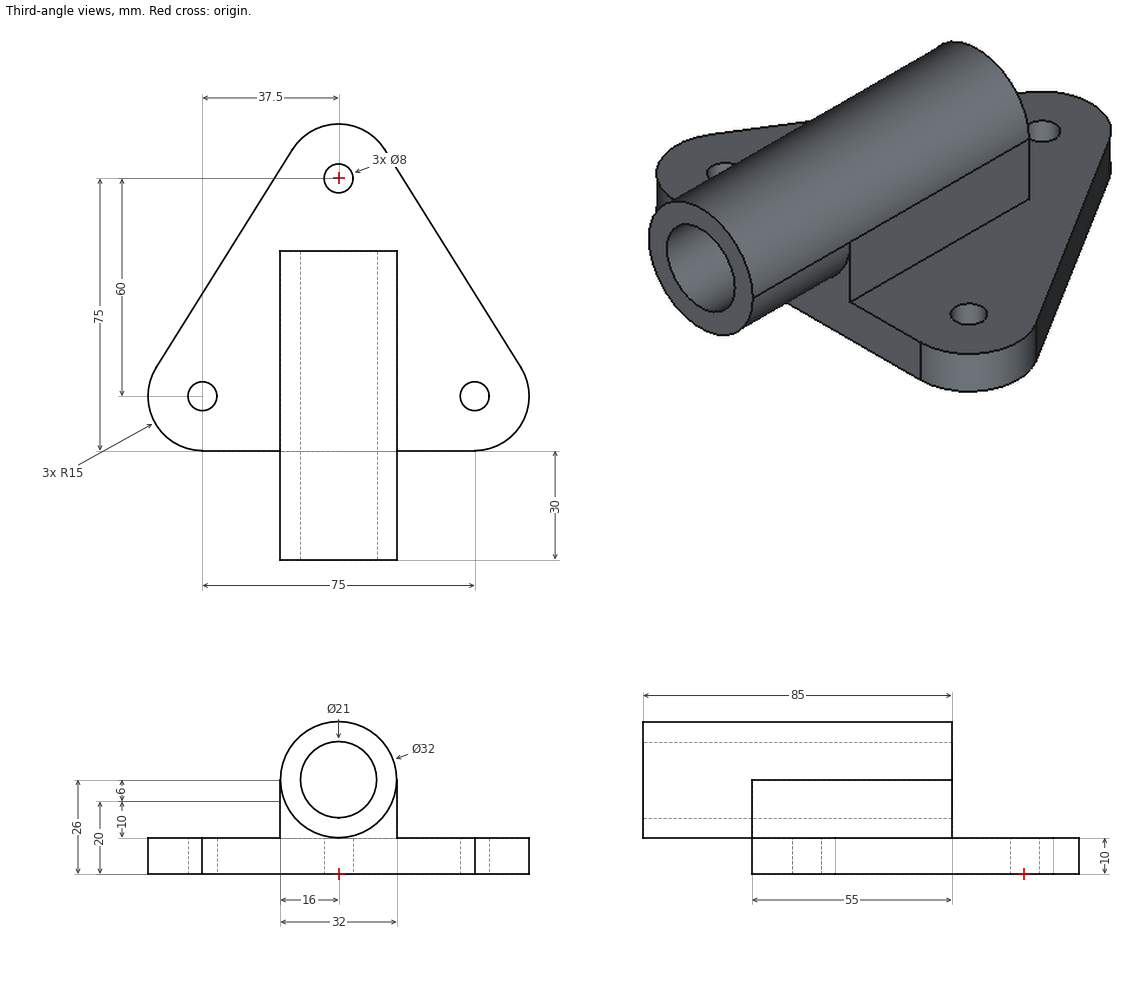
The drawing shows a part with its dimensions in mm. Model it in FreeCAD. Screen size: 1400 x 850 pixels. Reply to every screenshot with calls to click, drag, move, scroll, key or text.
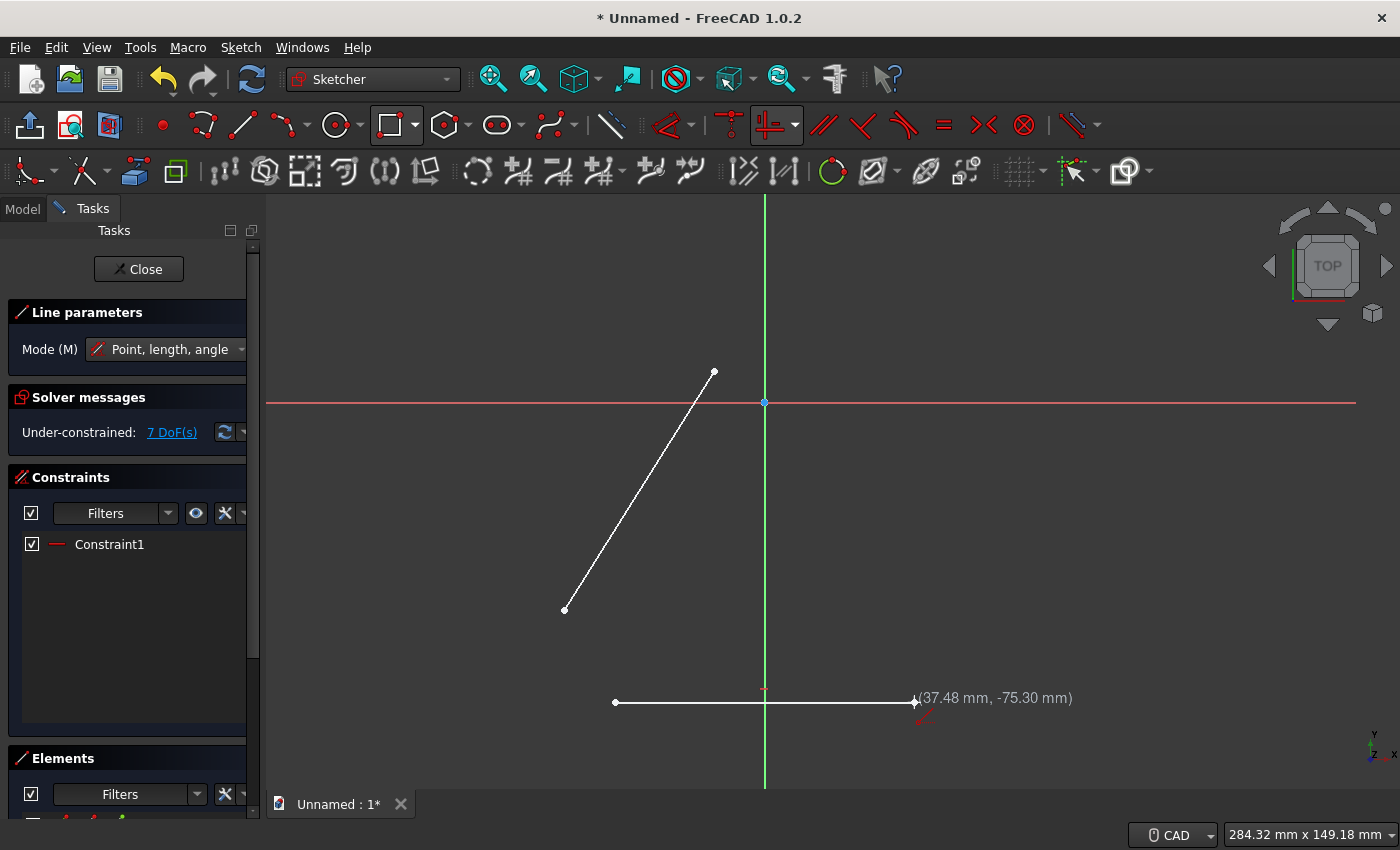
click(965, 610)
click(815, 371)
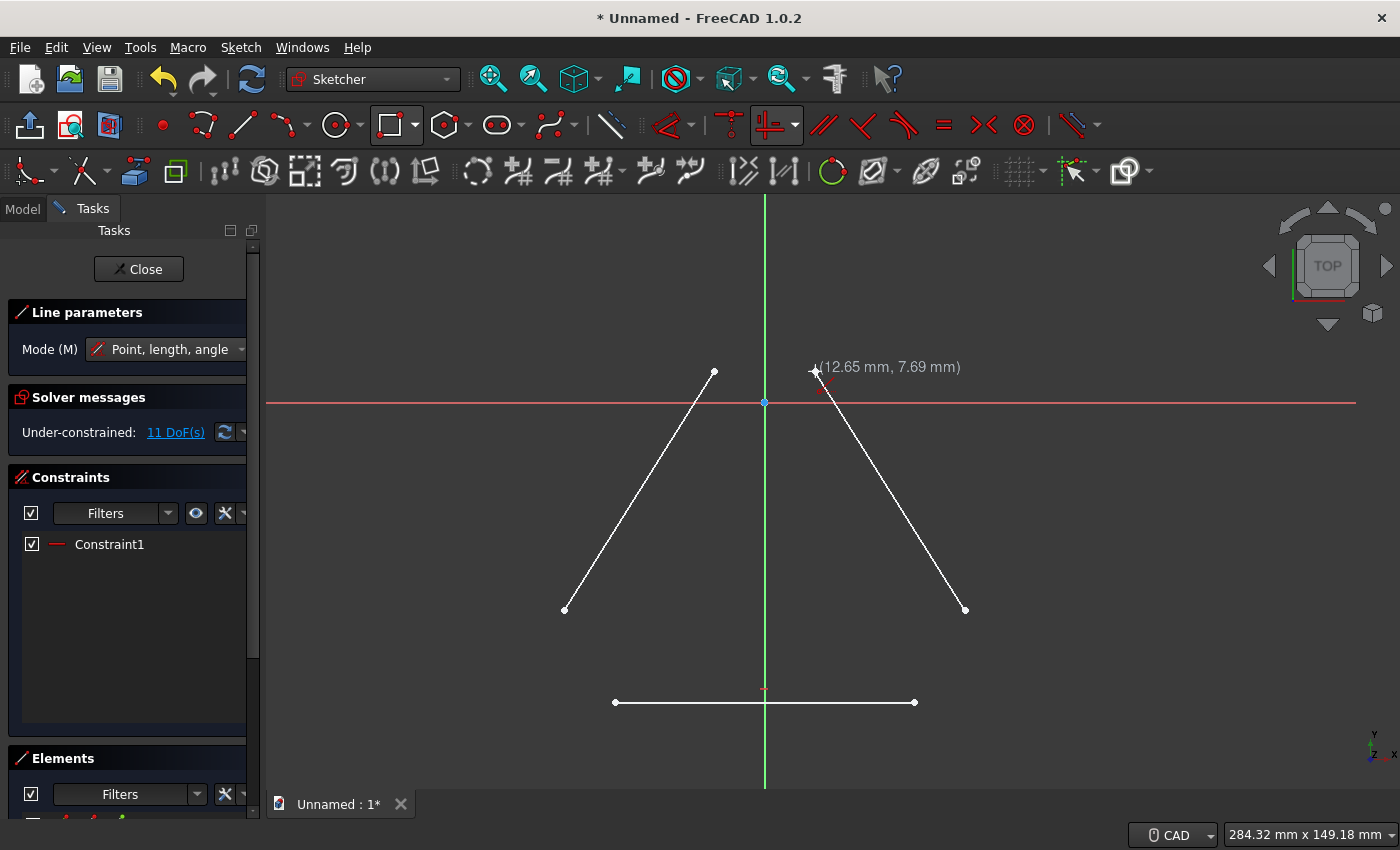
click(284, 126)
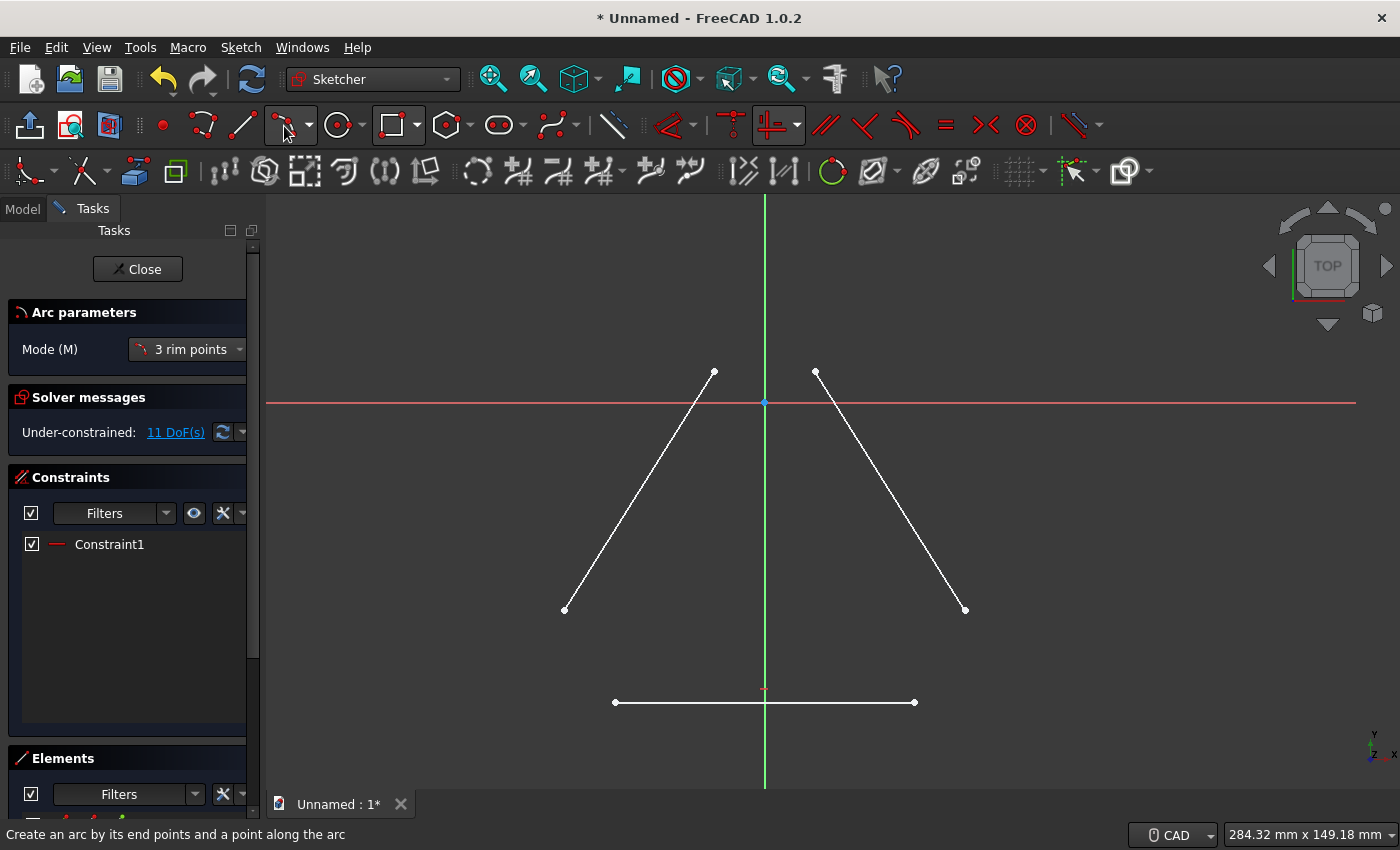
click(564, 611)
click(615, 703)
click(563, 671)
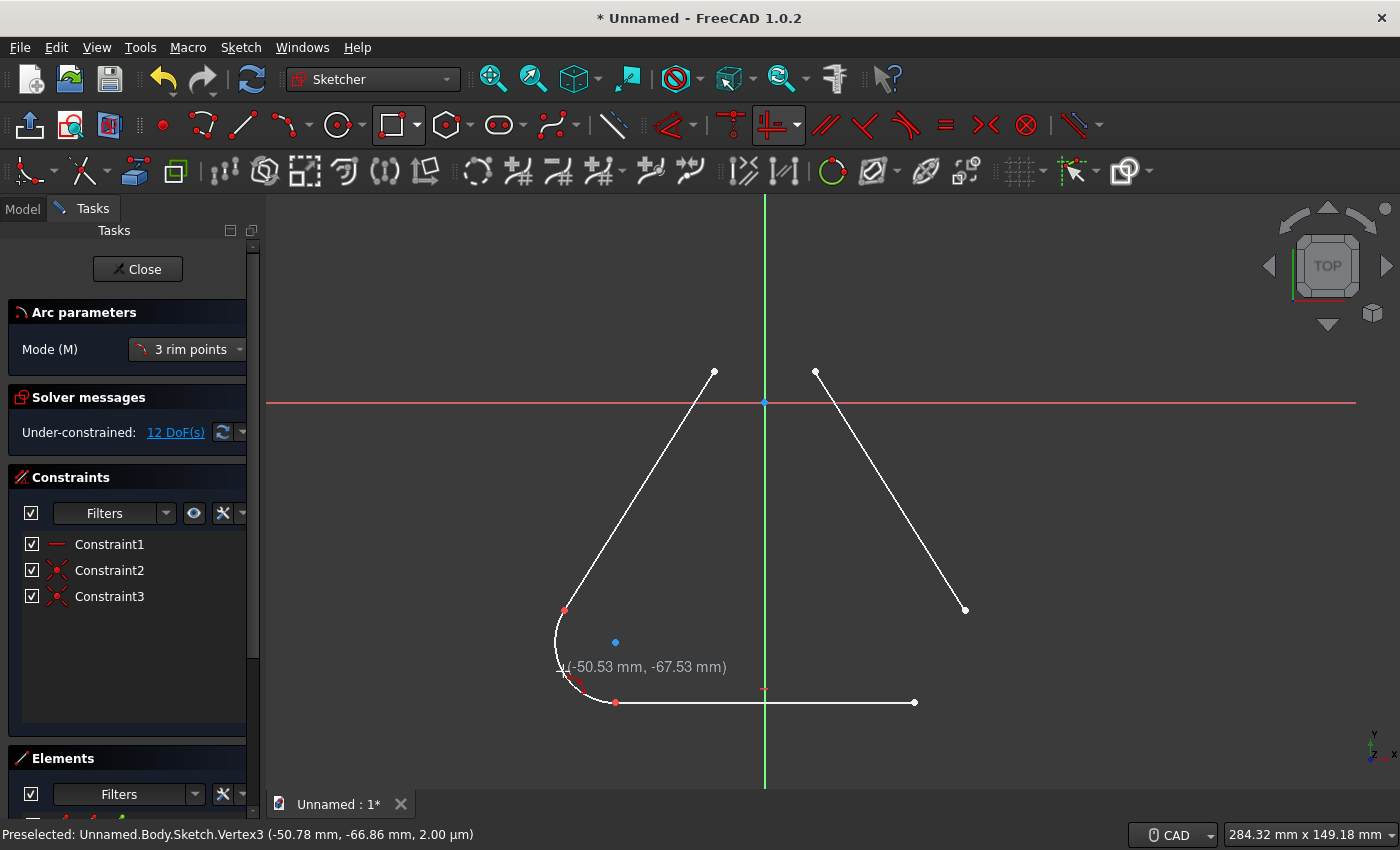
click(914, 703)
click(965, 611)
click(966, 671)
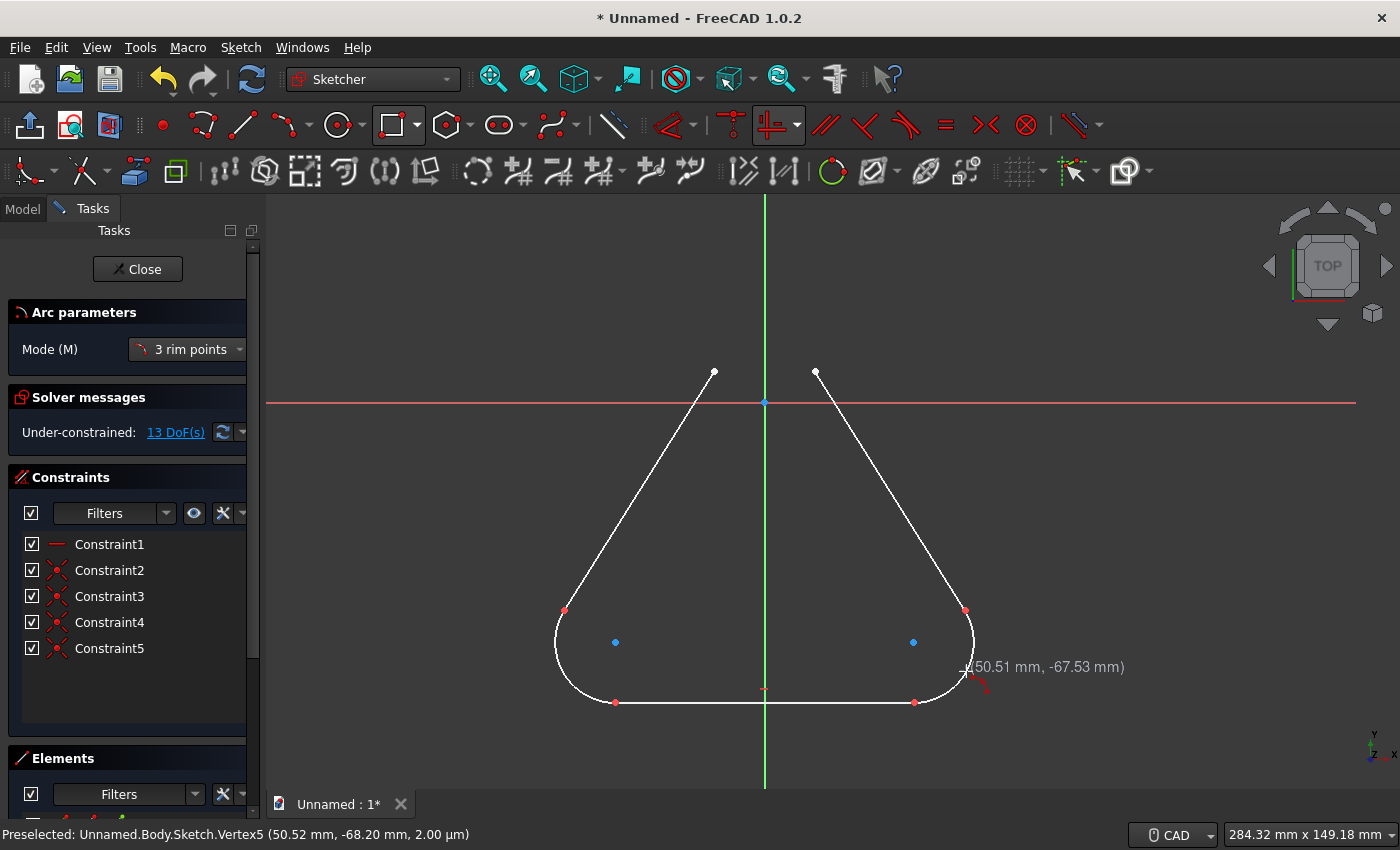
click(815, 372)
click(714, 372)
click(788, 348)
key(Escape)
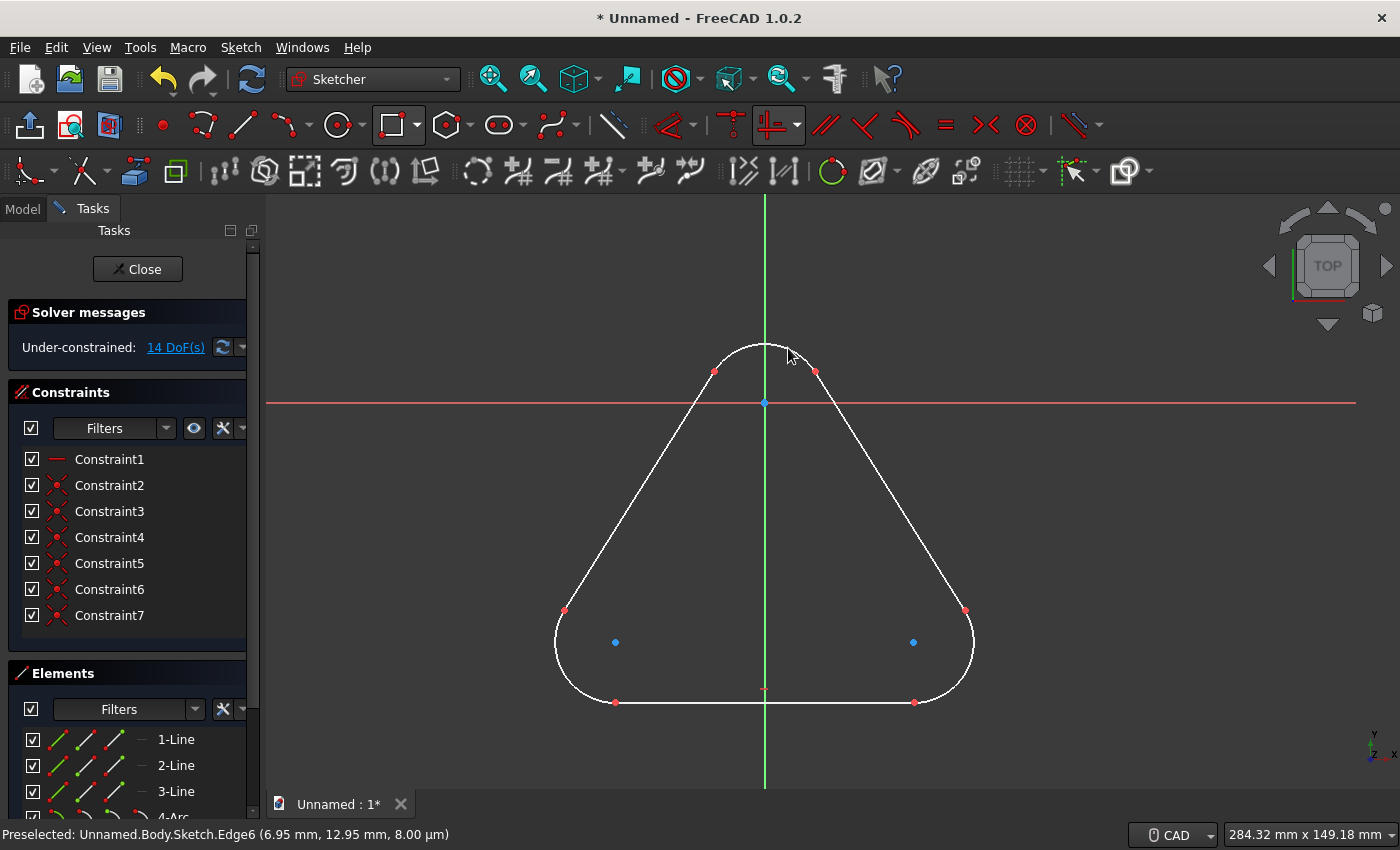
click(669, 444)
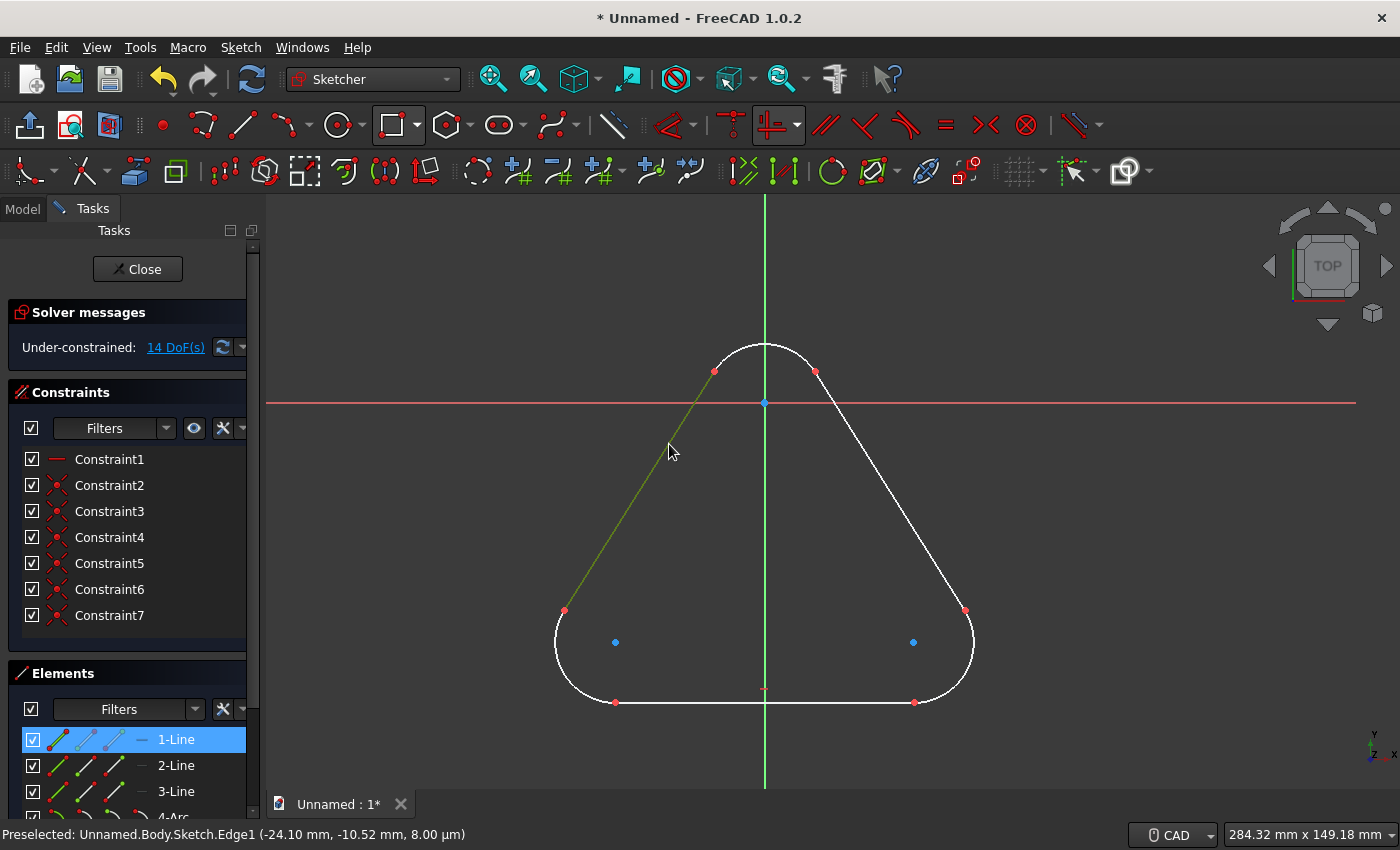
click(555, 648)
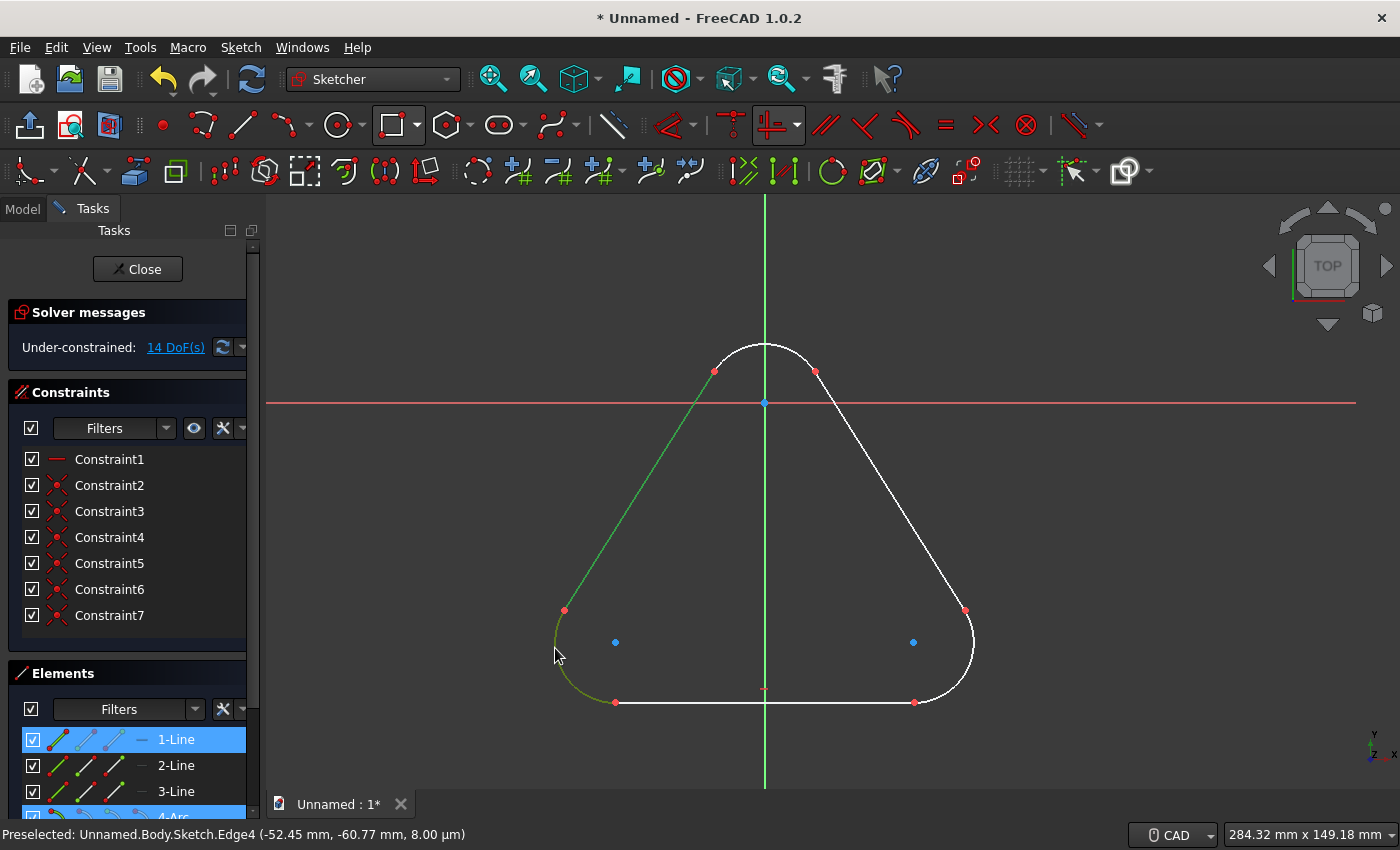
click(906, 126)